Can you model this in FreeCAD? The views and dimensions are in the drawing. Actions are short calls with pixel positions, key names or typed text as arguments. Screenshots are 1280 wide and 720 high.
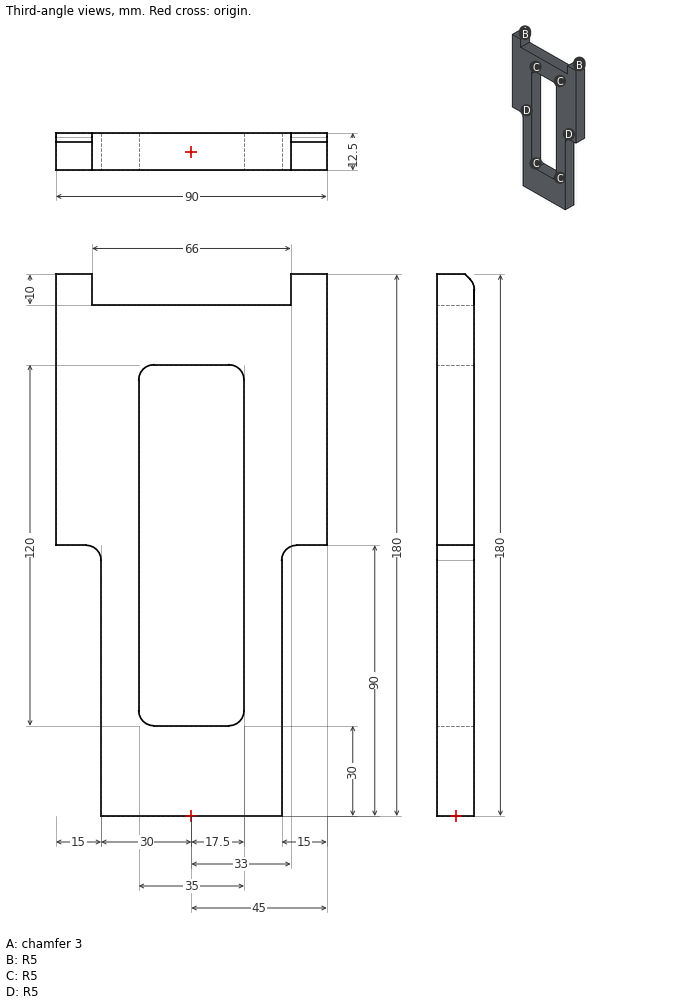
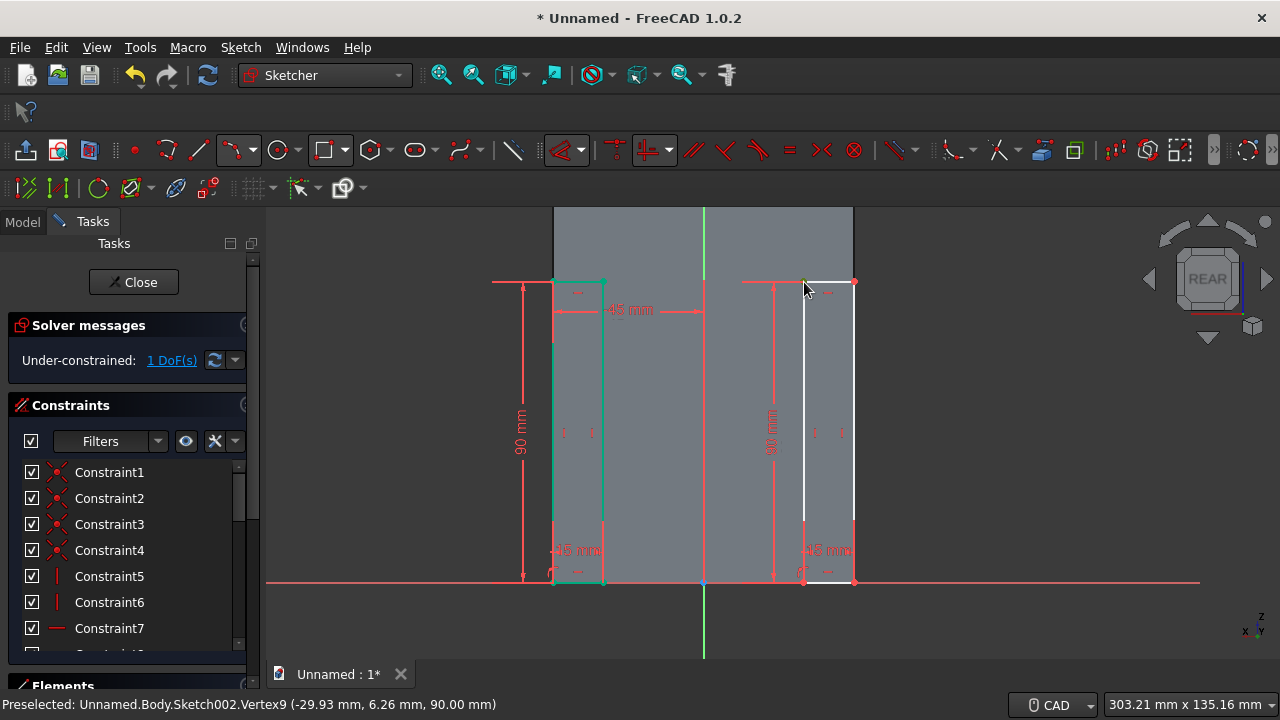
key(l)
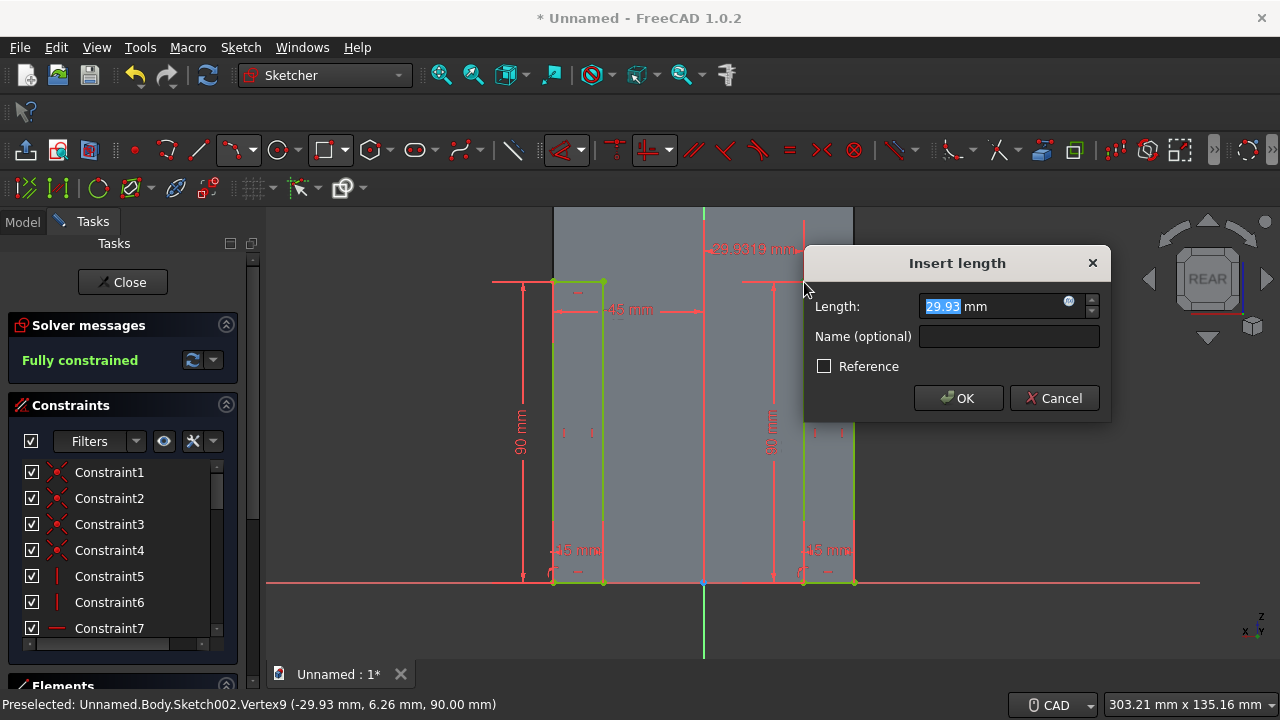
text(30)
key(Return)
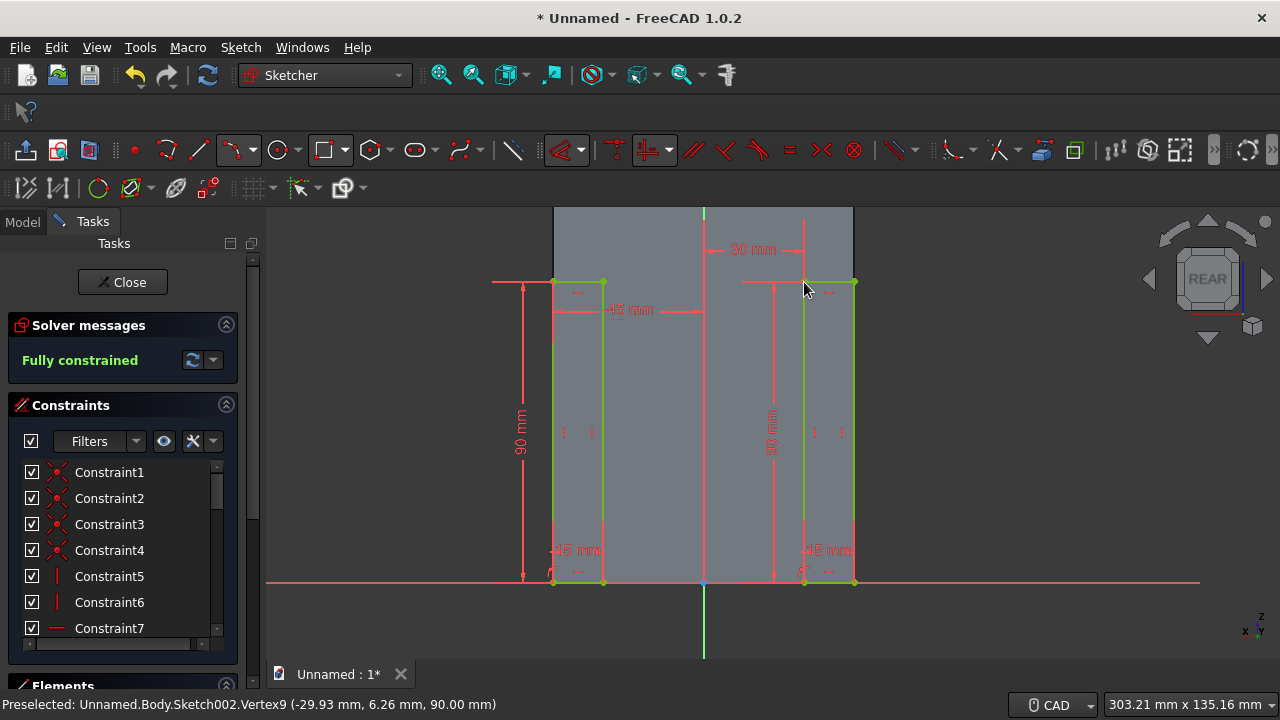
click(123, 282)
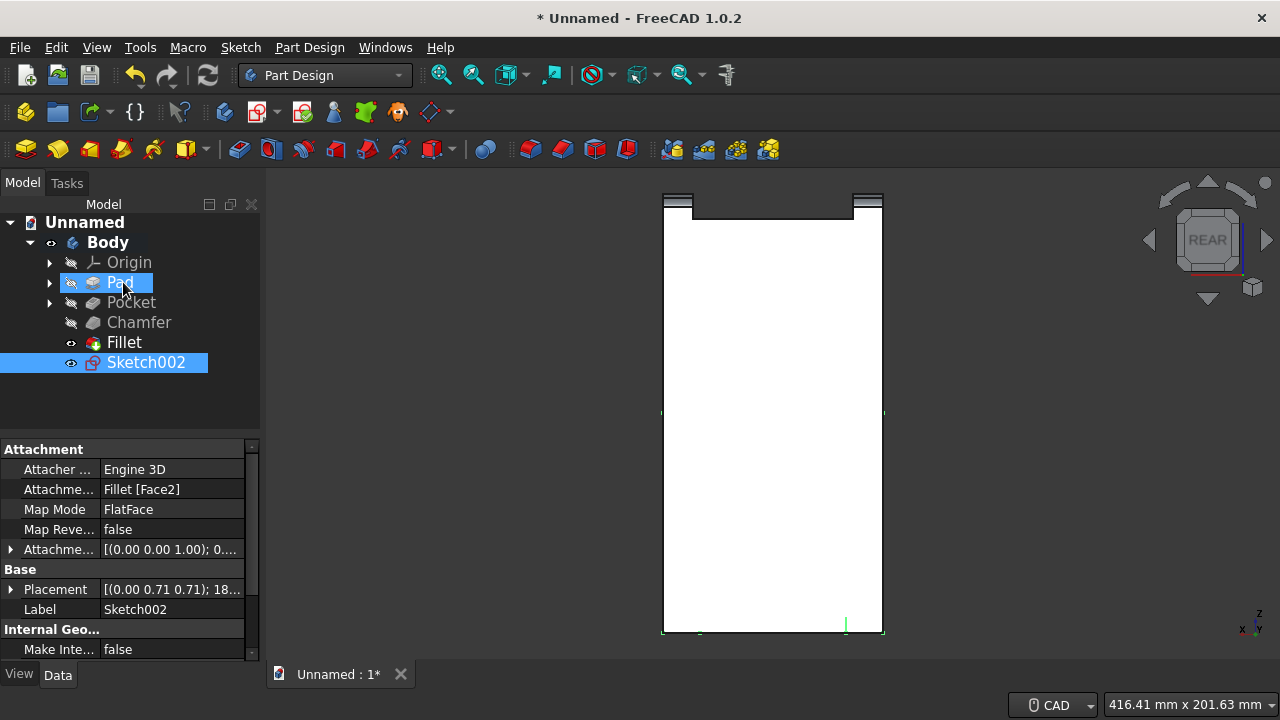
click(240, 150)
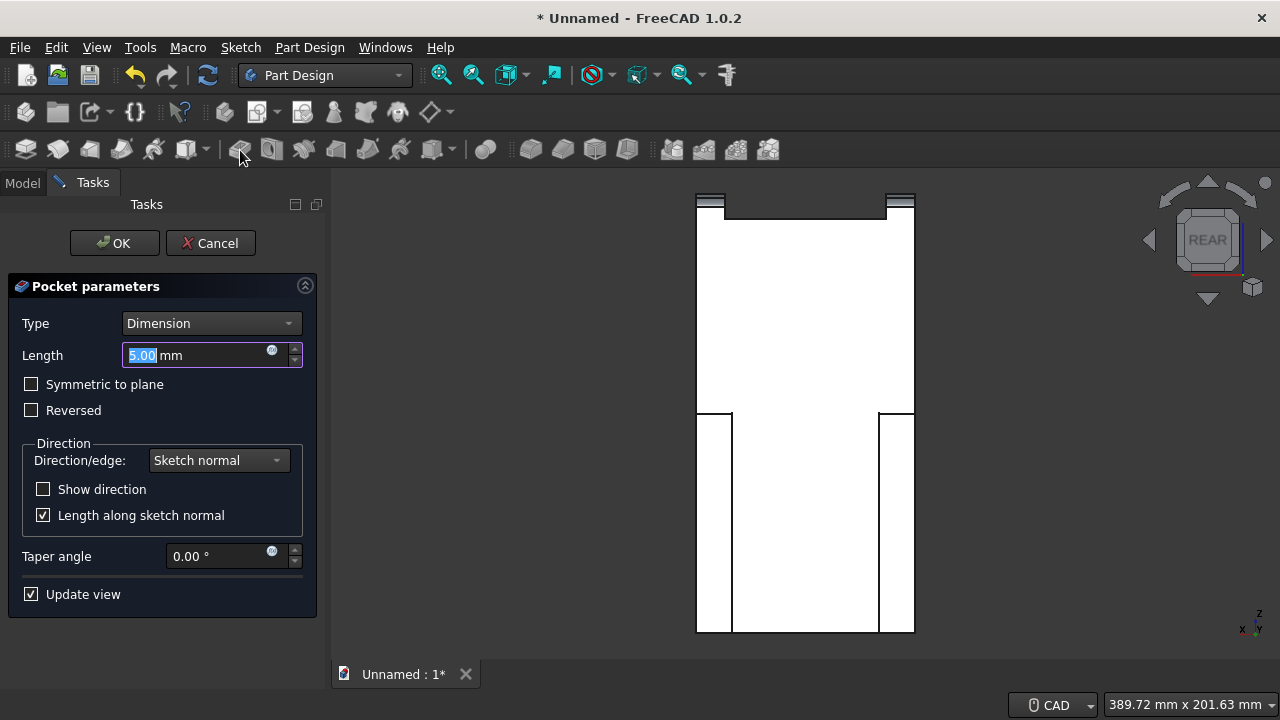
click(212, 324)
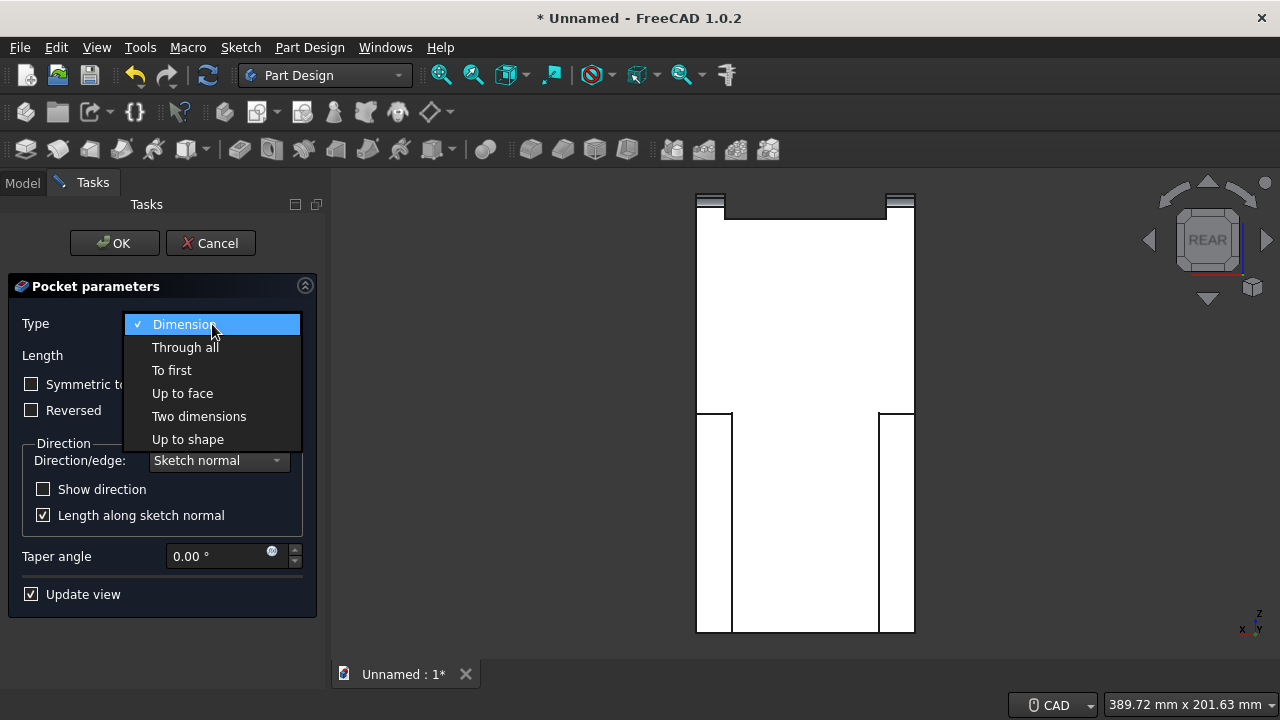
click(212, 348)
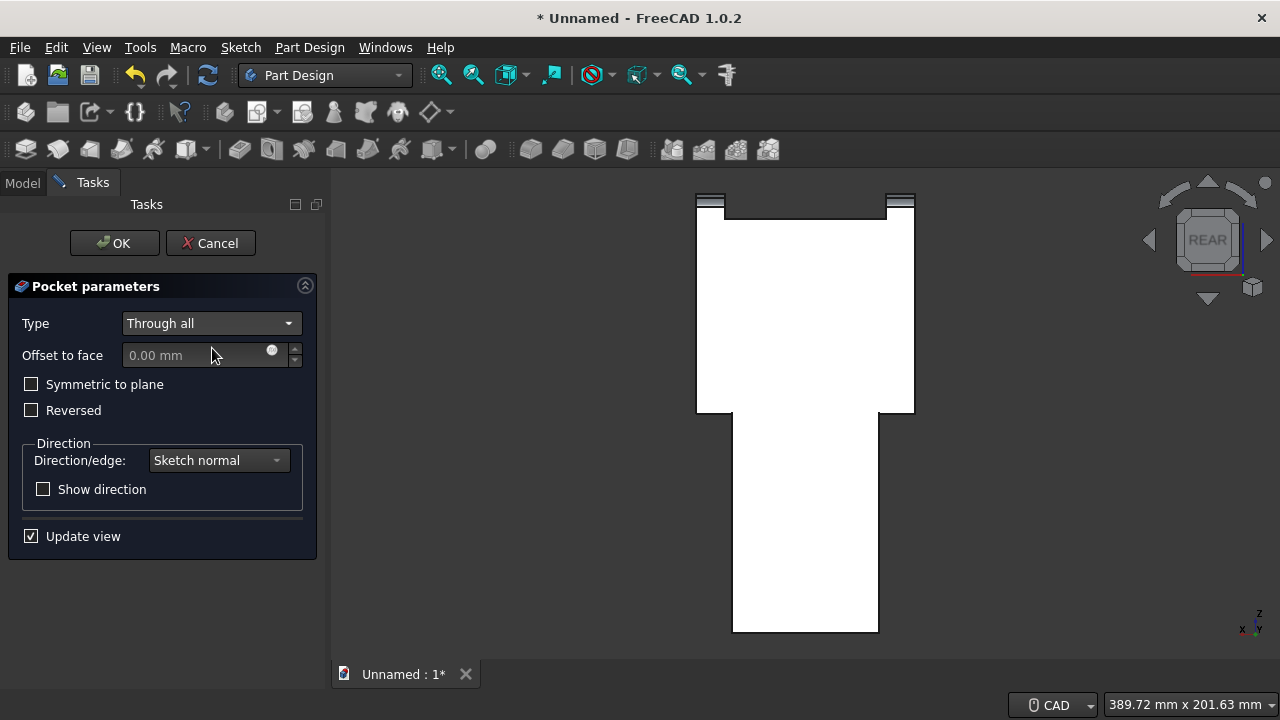
click(115, 243)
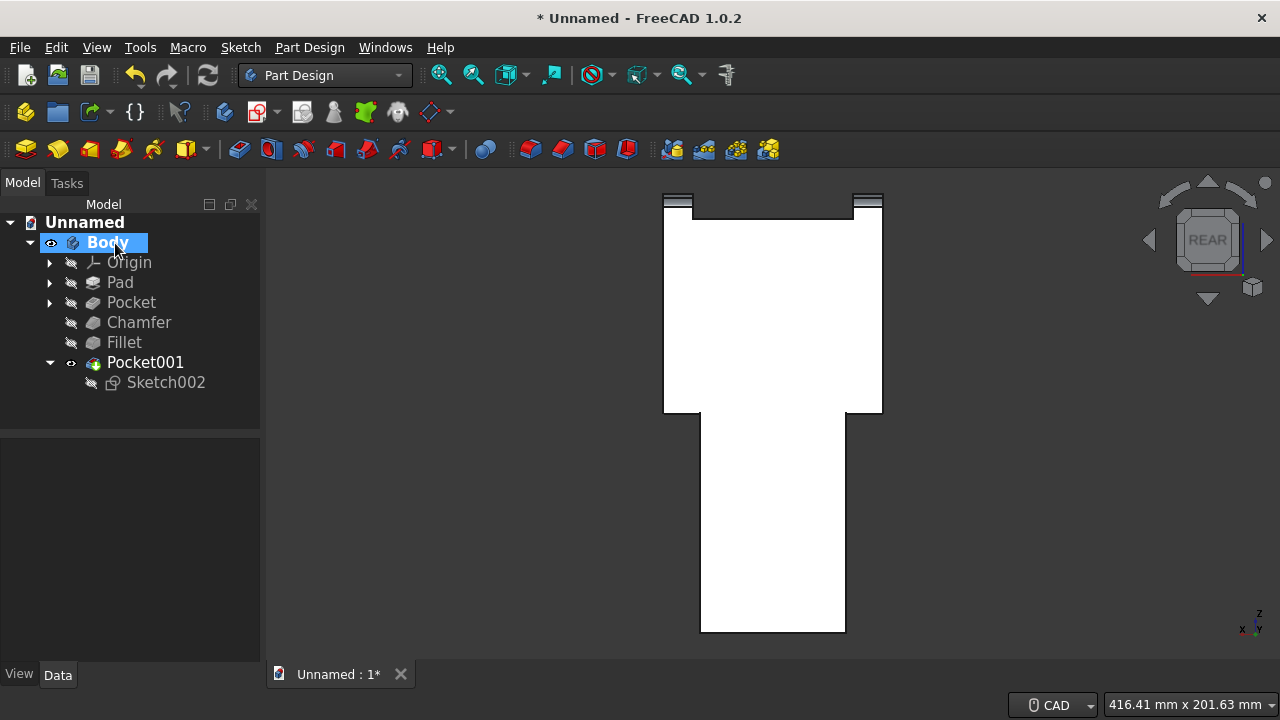
click(773, 358)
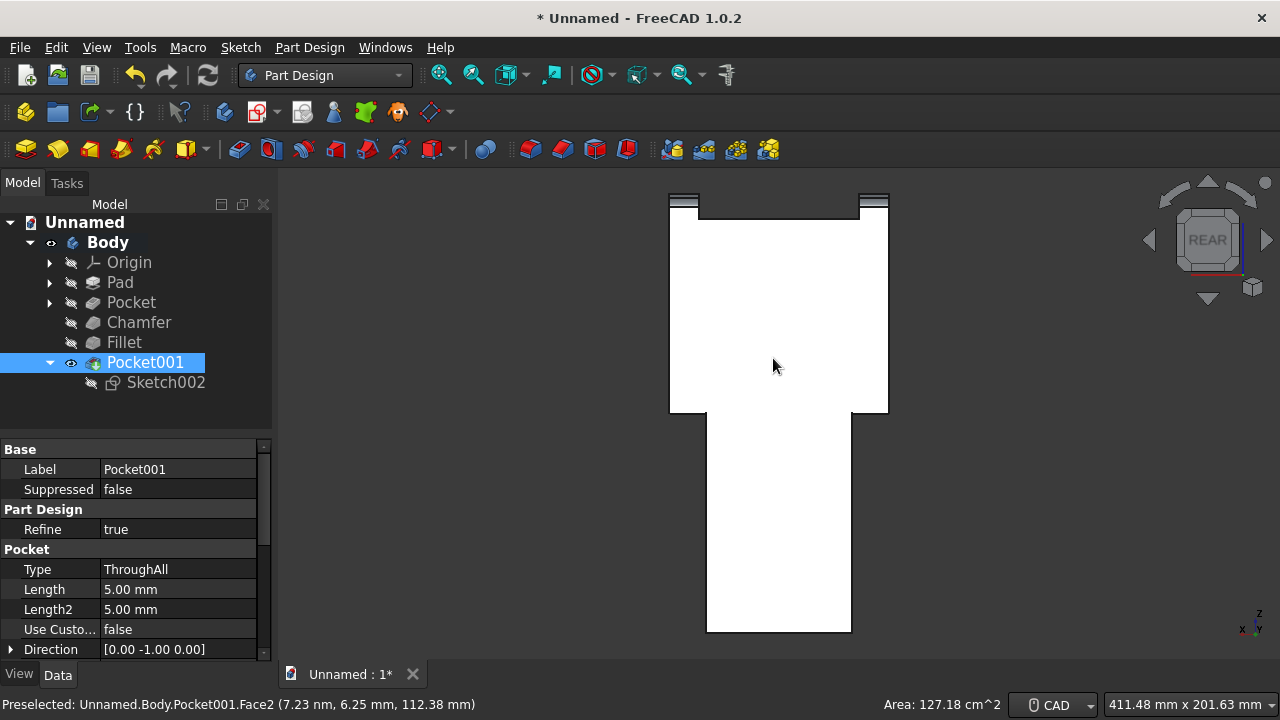
click(258, 112)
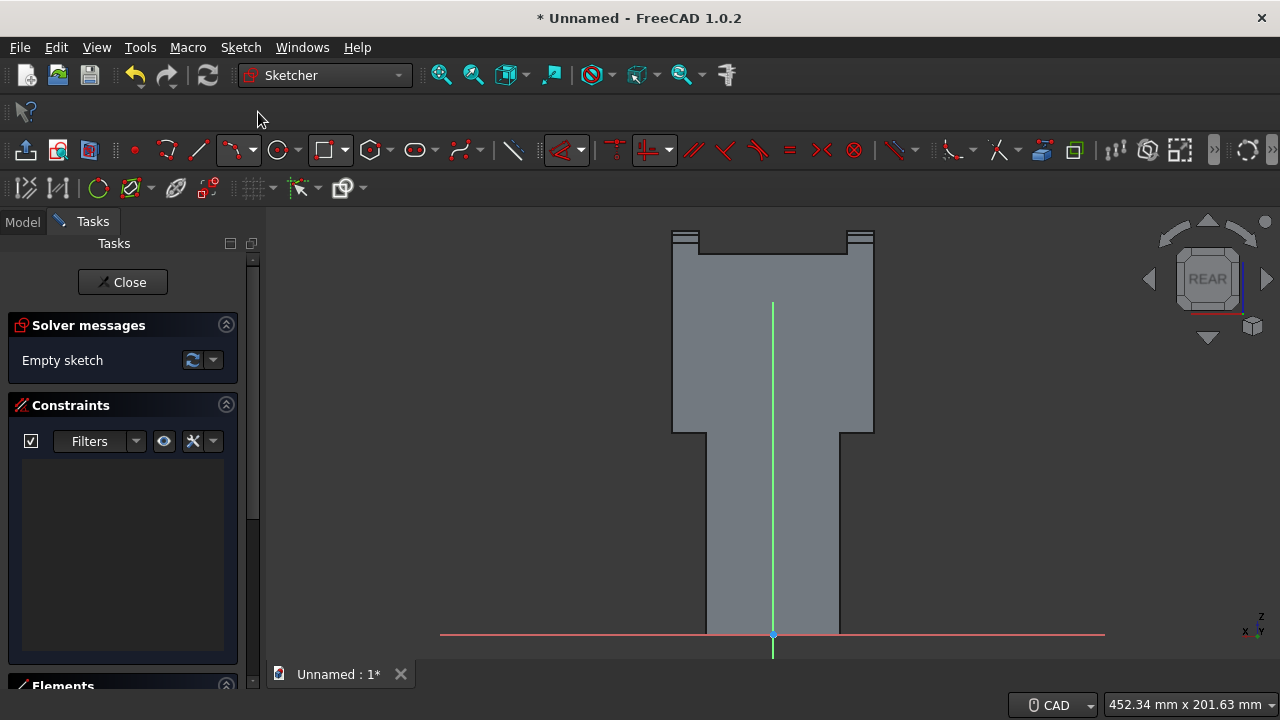
scroll(395, 281, down, 1)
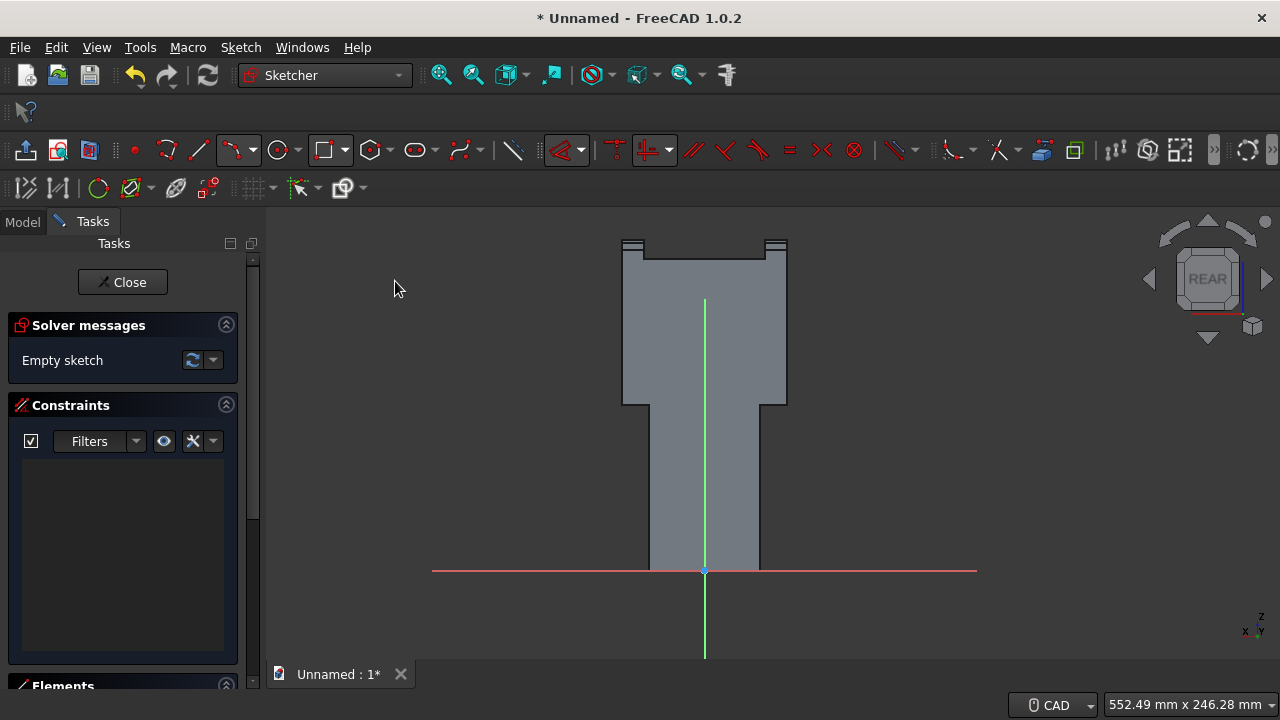
click(324, 150)